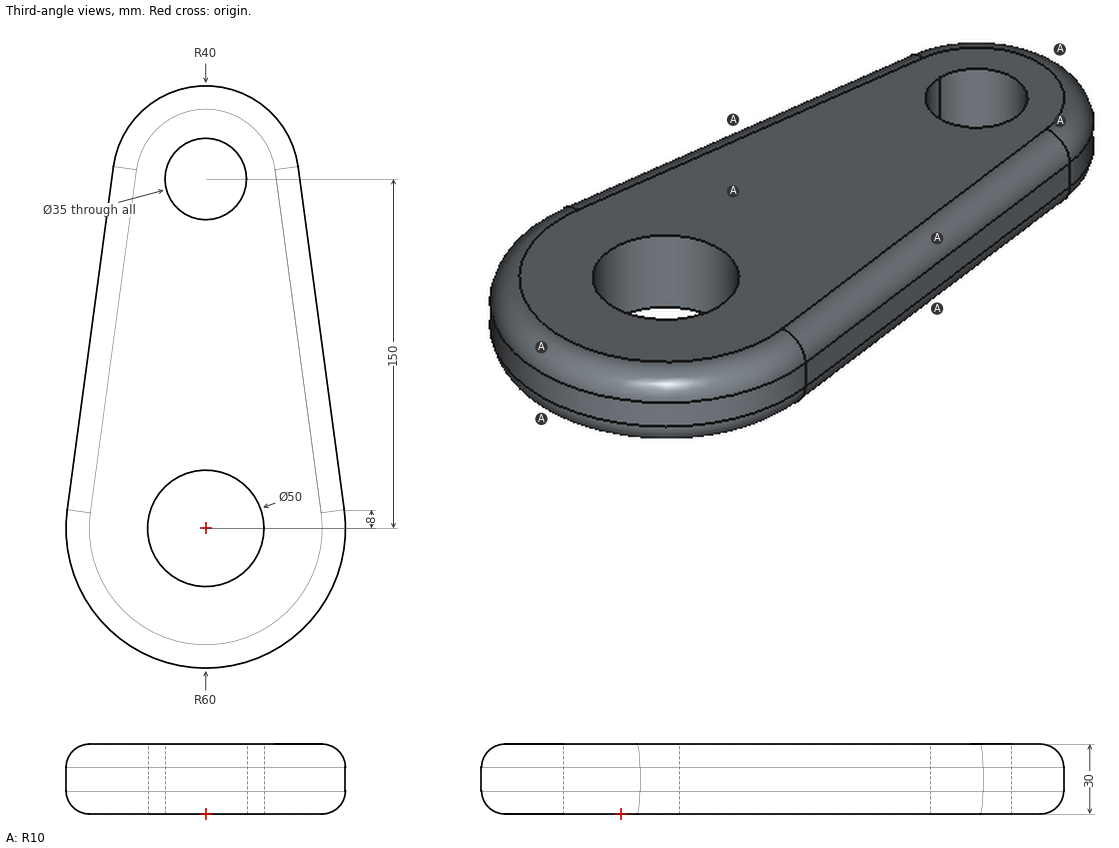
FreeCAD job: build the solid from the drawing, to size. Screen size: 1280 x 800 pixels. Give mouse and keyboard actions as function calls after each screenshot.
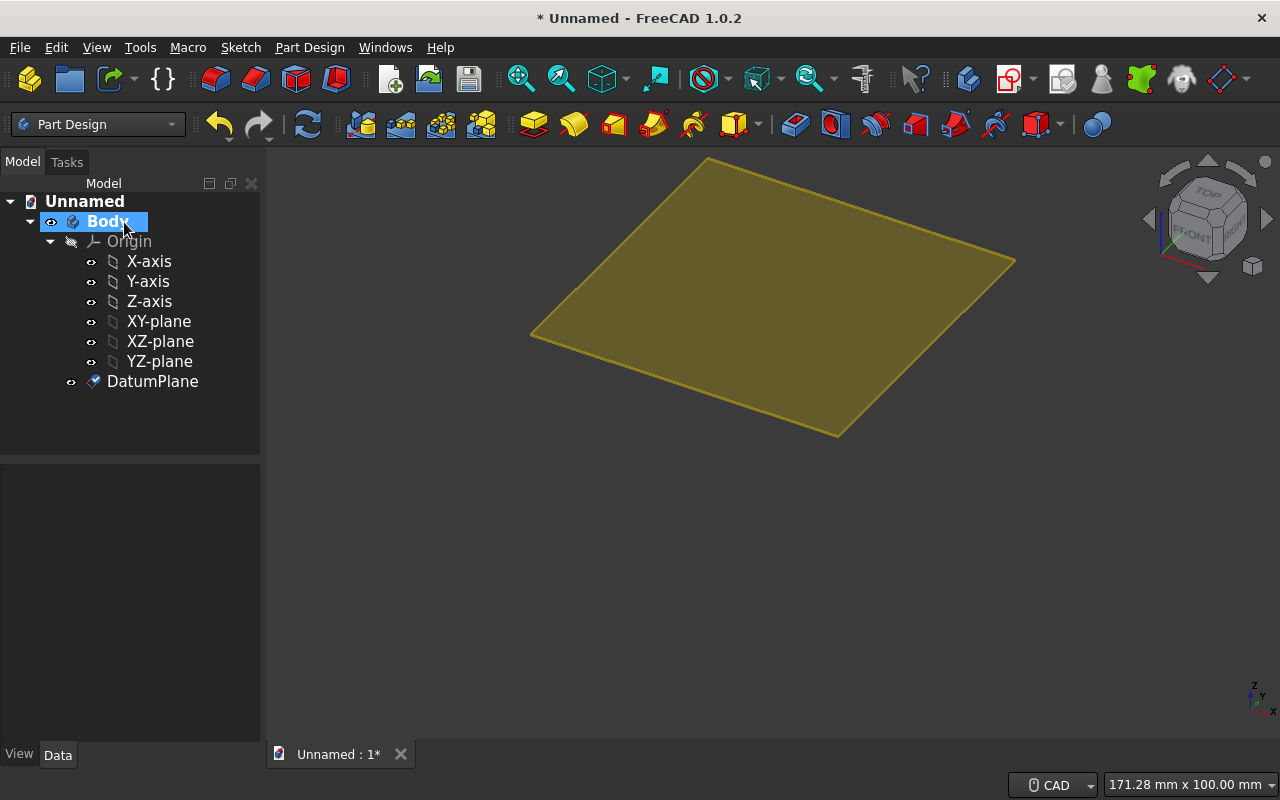
click(116, 382)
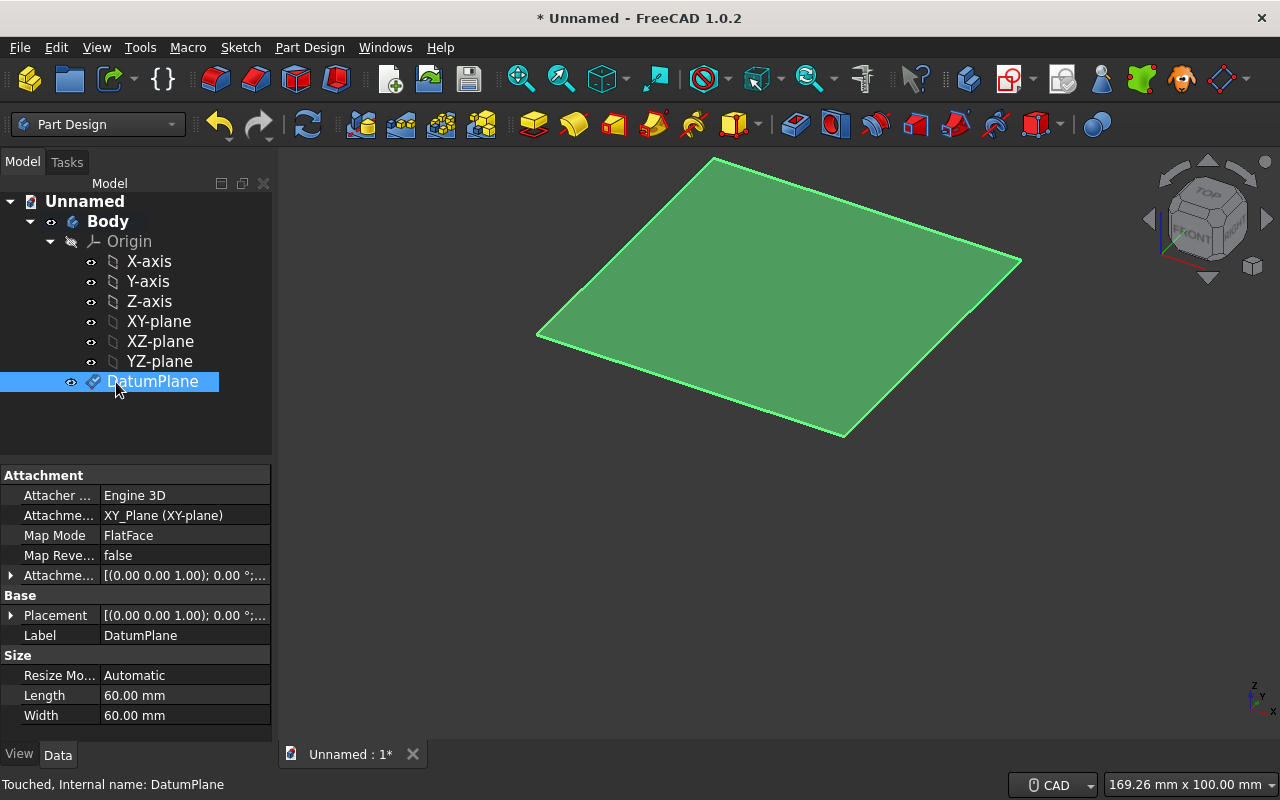
click(1010, 80)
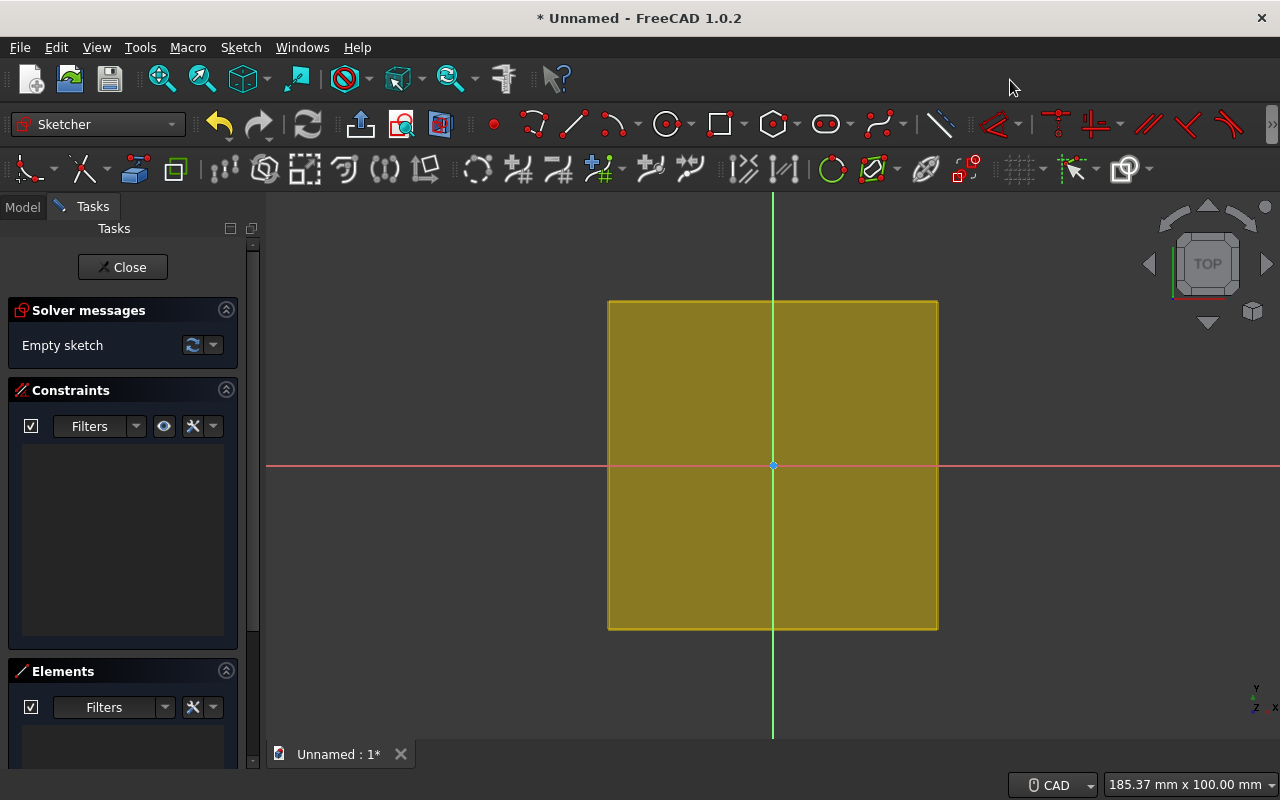
scroll(682, 582, down, 7)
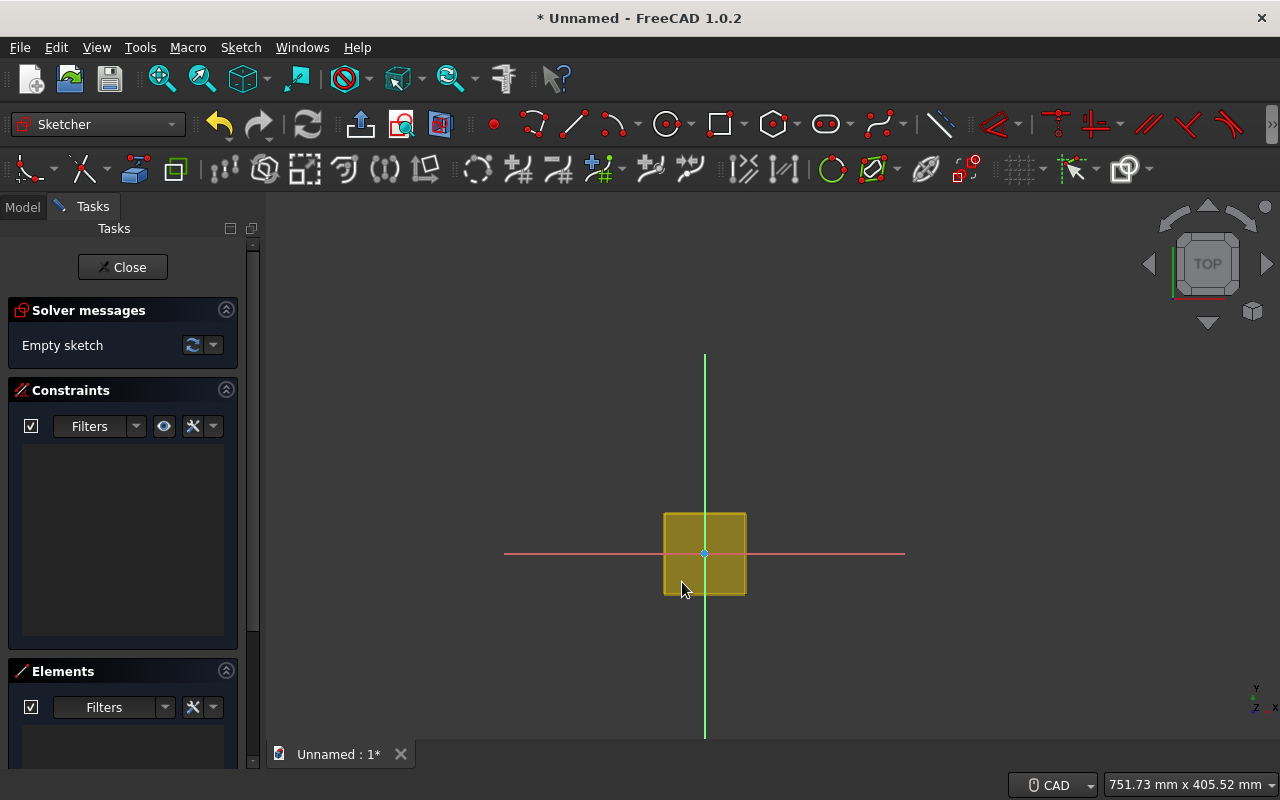
click(574, 124)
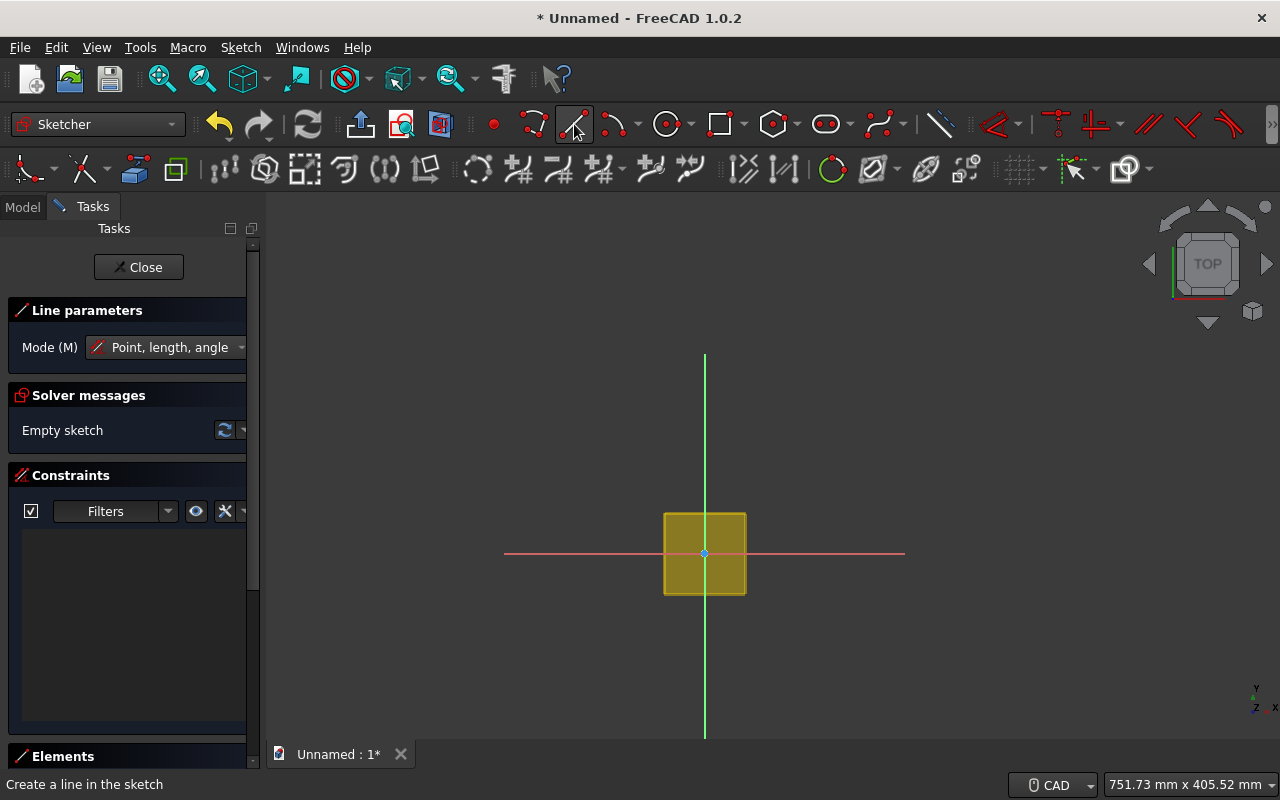
scroll(785, 543, up, 2)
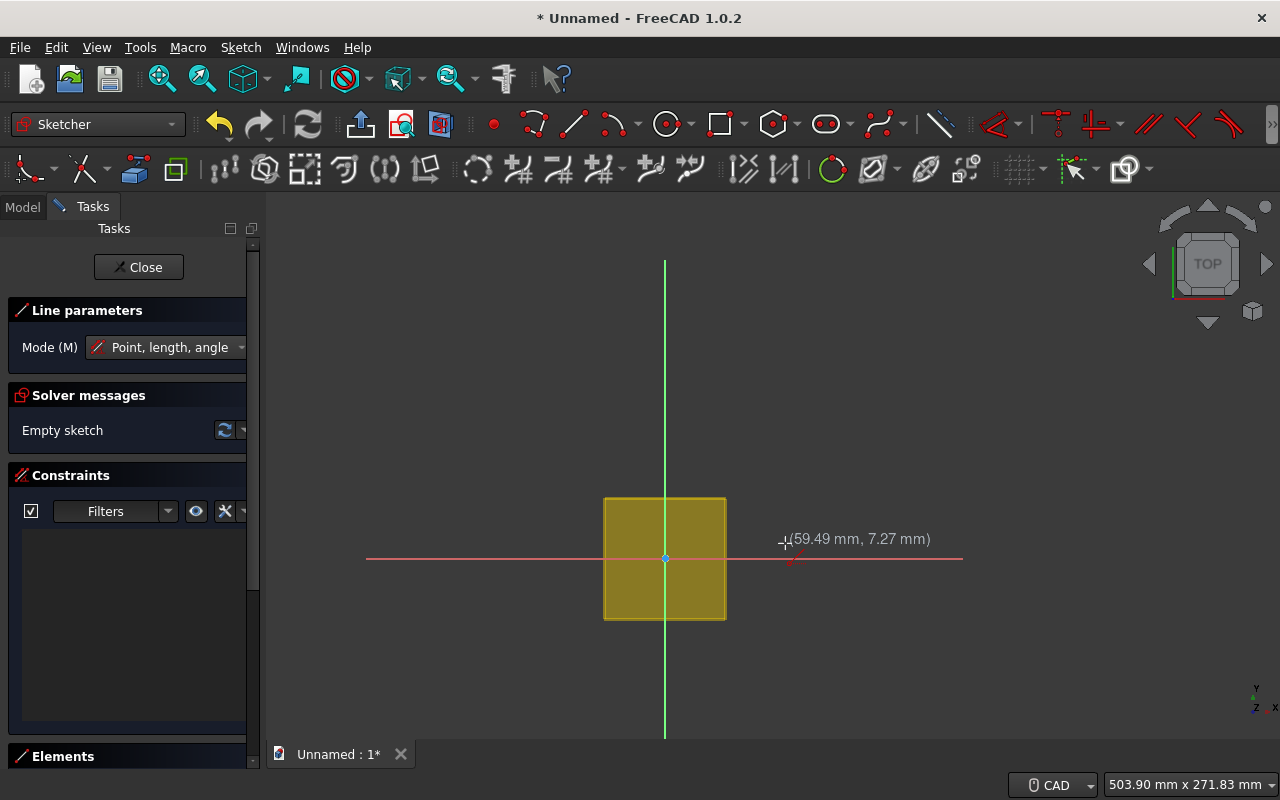
click(785, 543)
click(745, 246)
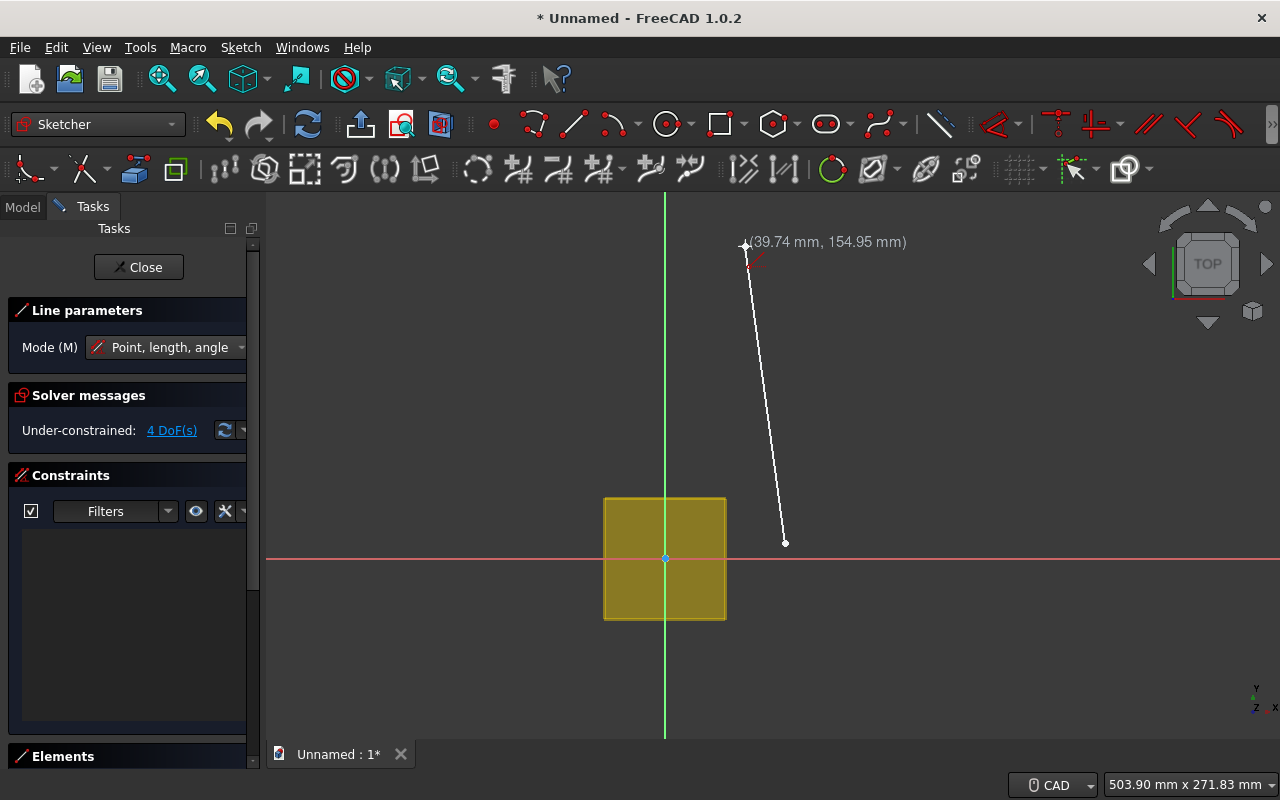
click(585, 246)
click(545, 543)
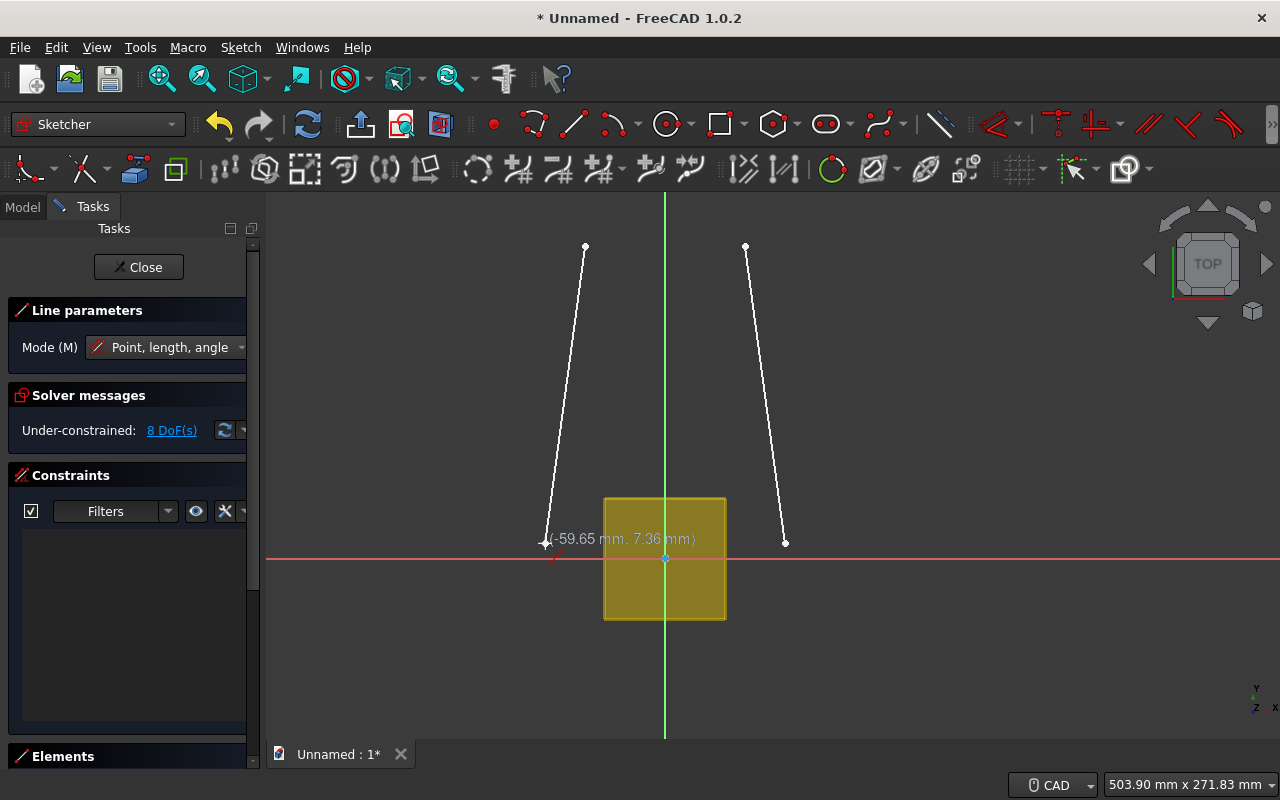
click(640, 124)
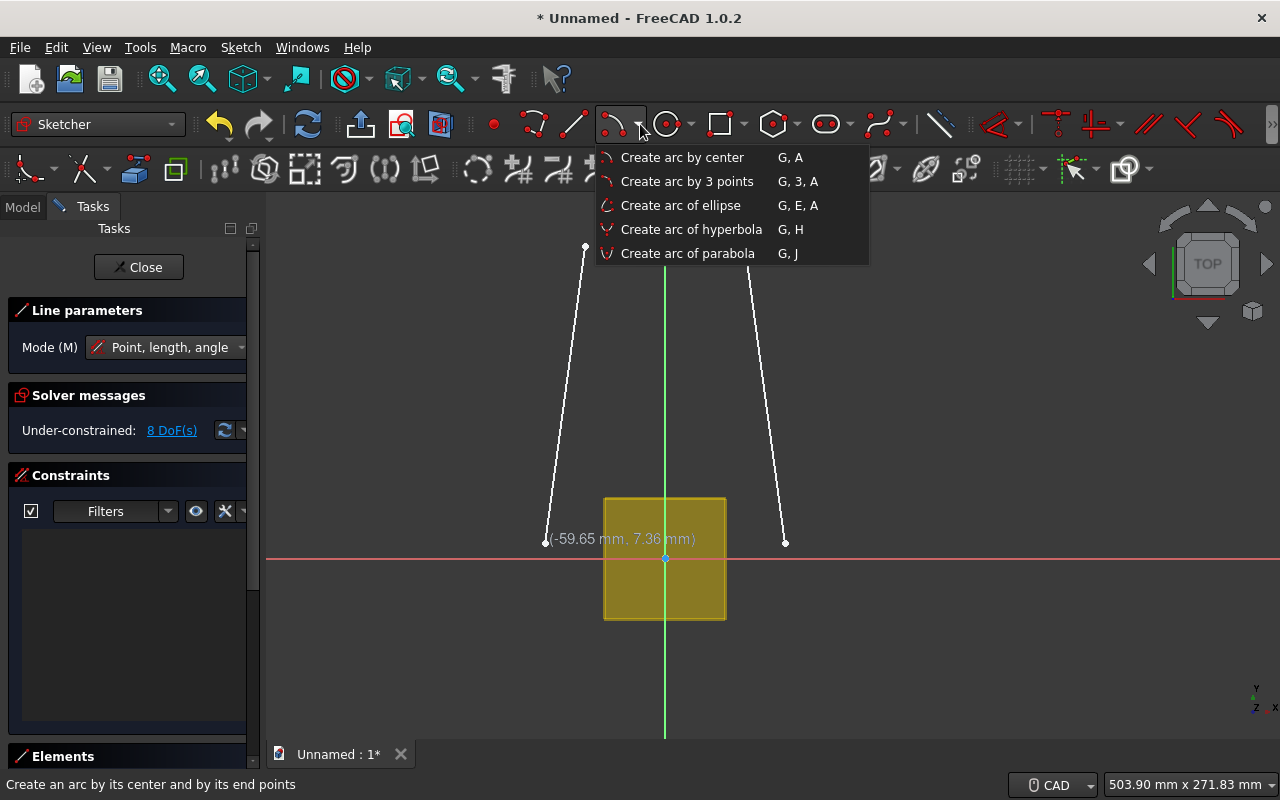
click(732, 181)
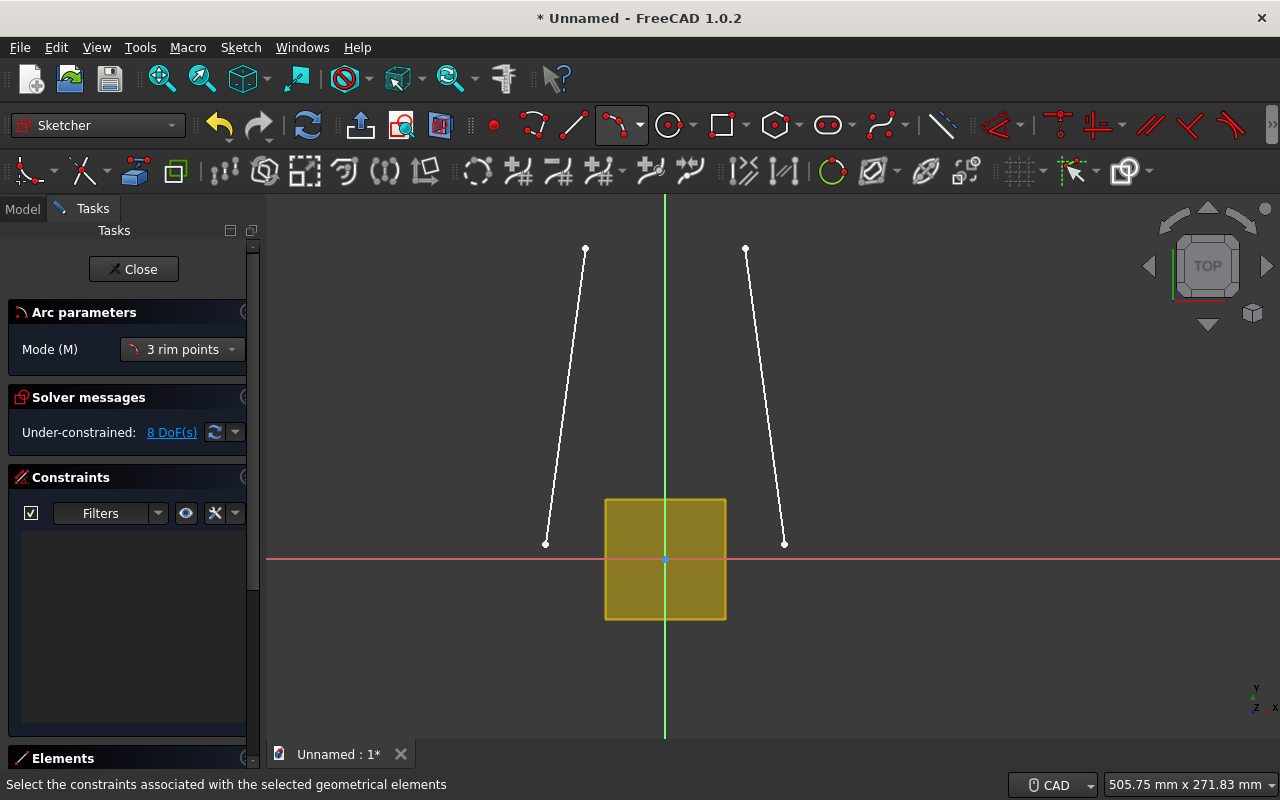
click(745, 249)
click(586, 249)